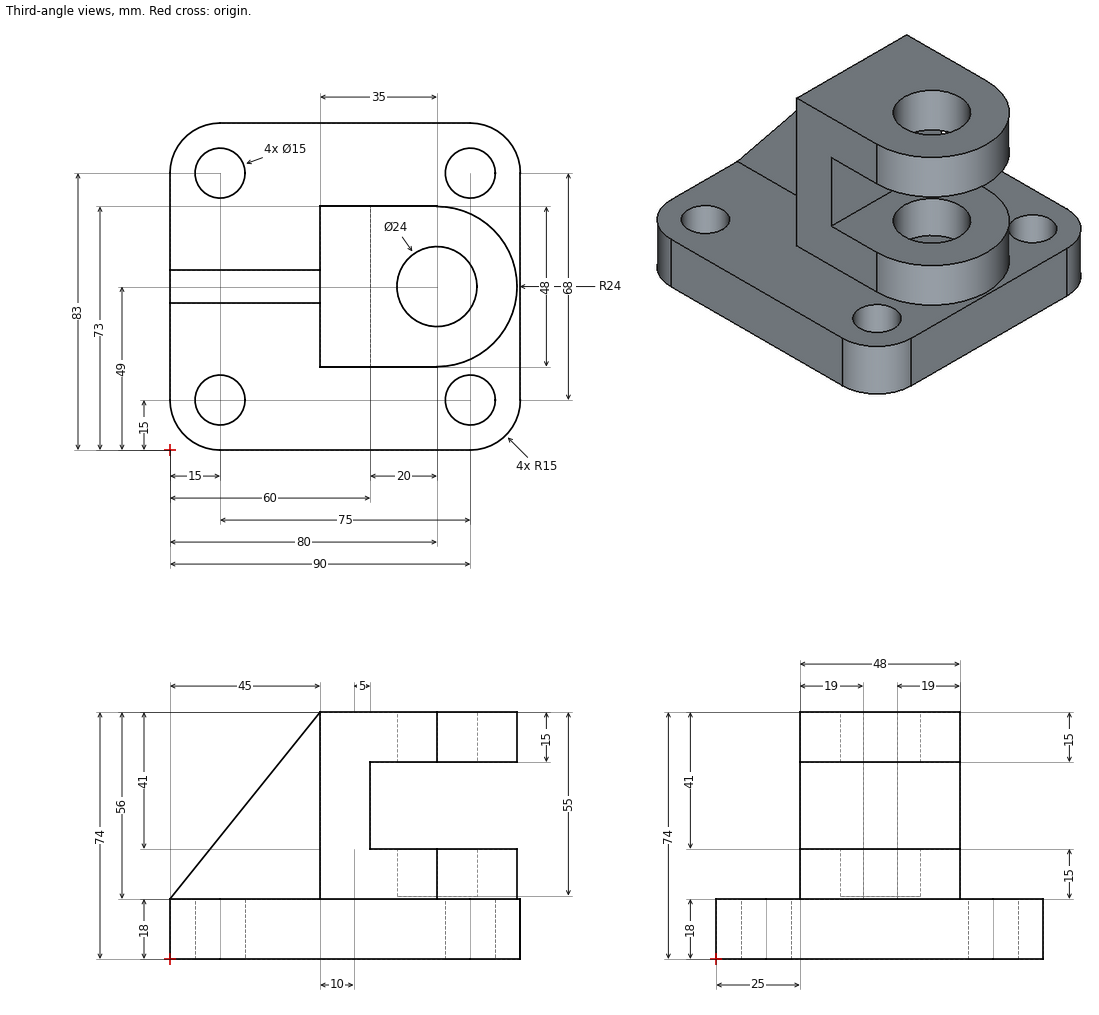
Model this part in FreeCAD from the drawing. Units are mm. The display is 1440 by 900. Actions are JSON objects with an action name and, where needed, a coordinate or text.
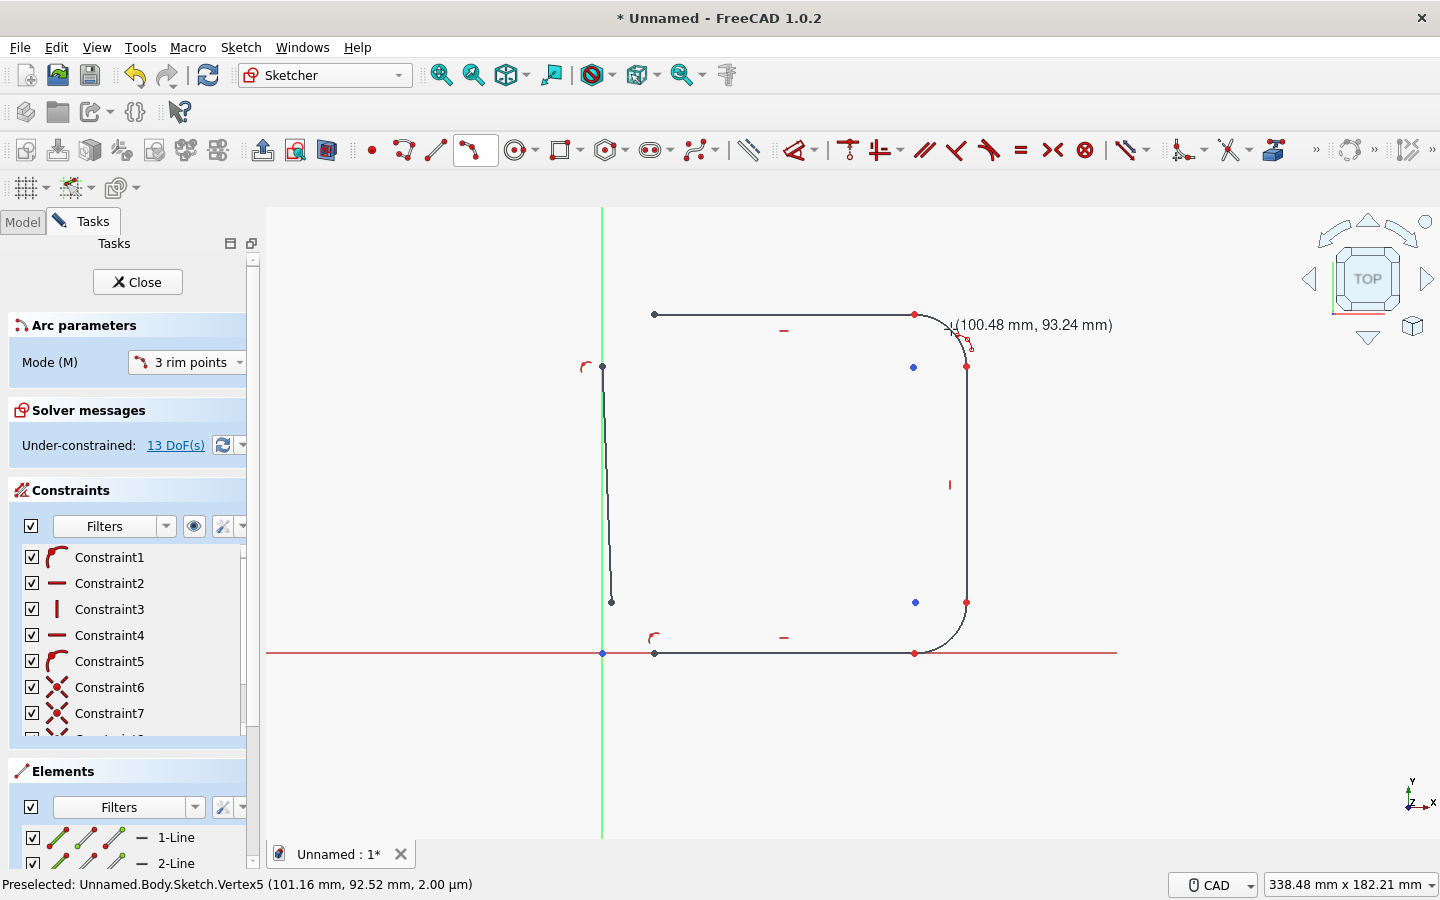
{"action": "left_click", "coordinate": [655, 315]}
{"action": "left_click", "coordinate": [602, 366]}
{"action": "left_click", "coordinate": [618, 329]}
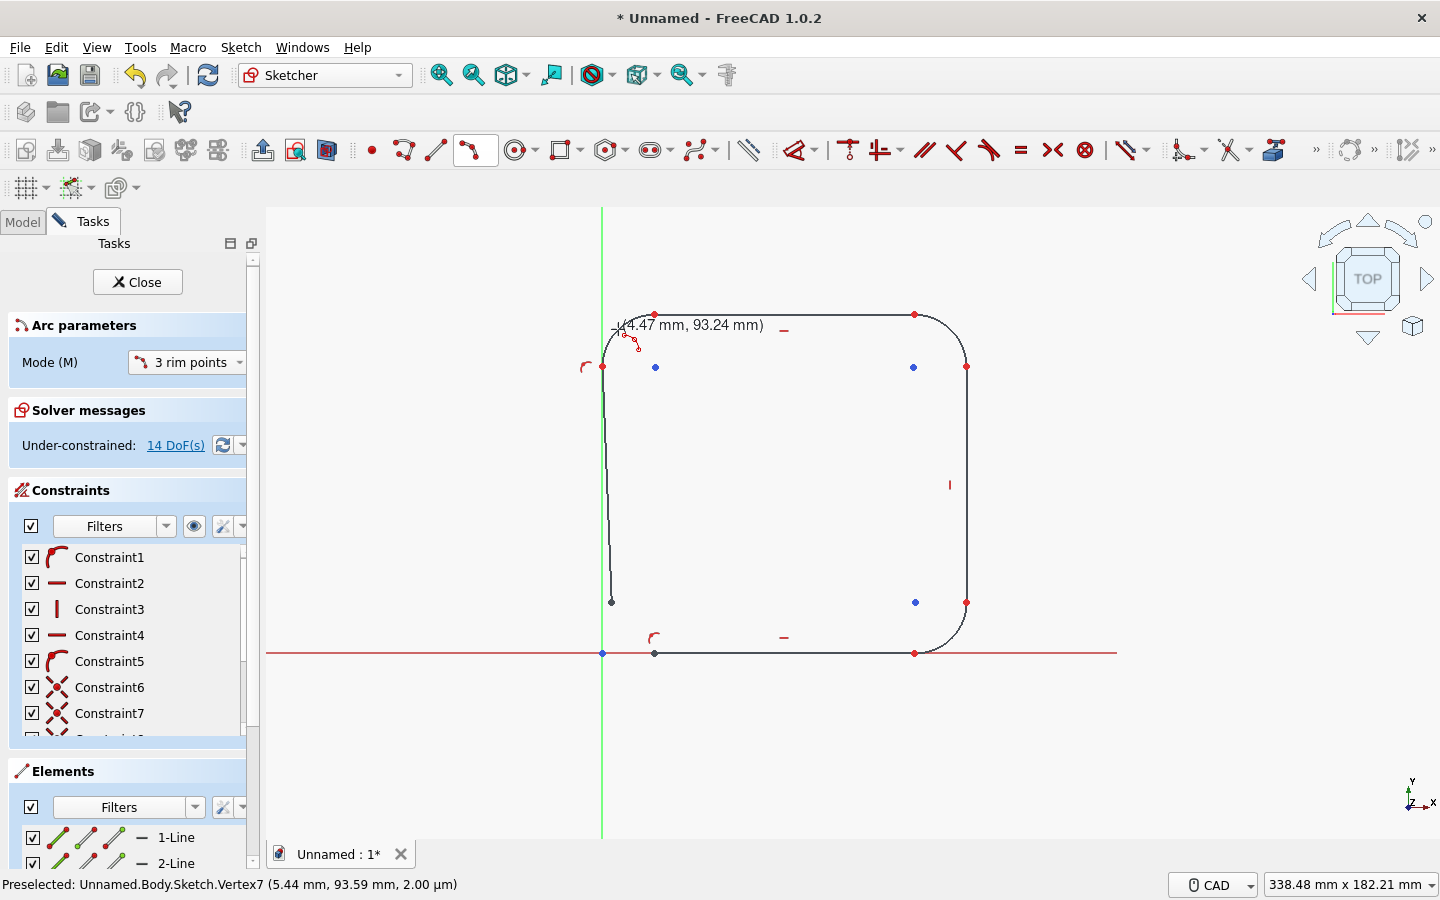
{"action": "left_click", "coordinate": [612, 603]}
{"action": "left_click", "coordinate": [655, 653]}
{"action": "left_click", "coordinate": [618, 638]}
{"action": "key", "text": "Escape"}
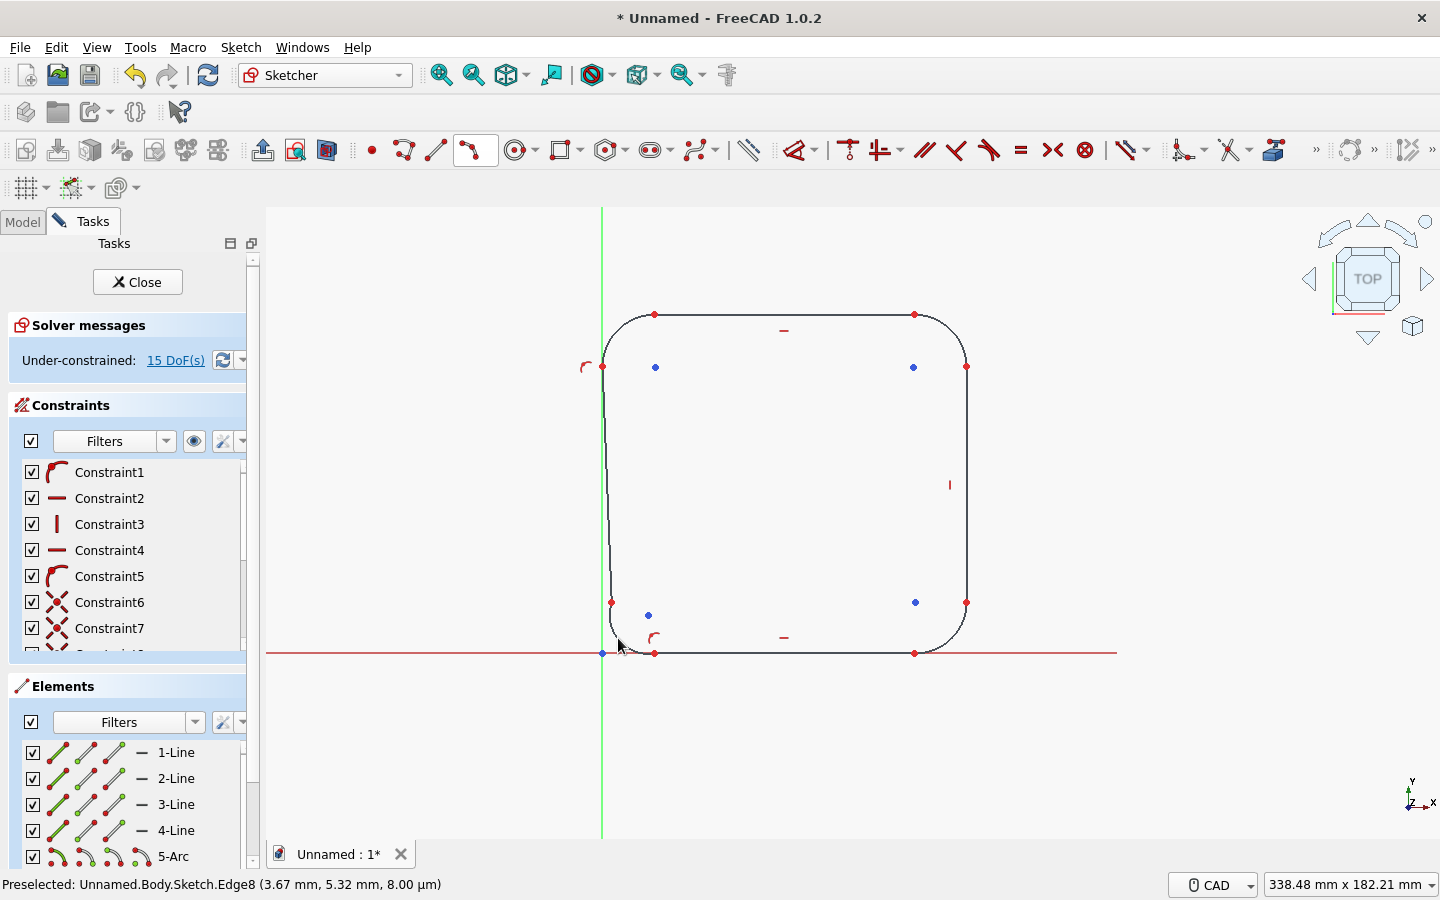
{"action": "left_click", "coordinate": [733, 653]}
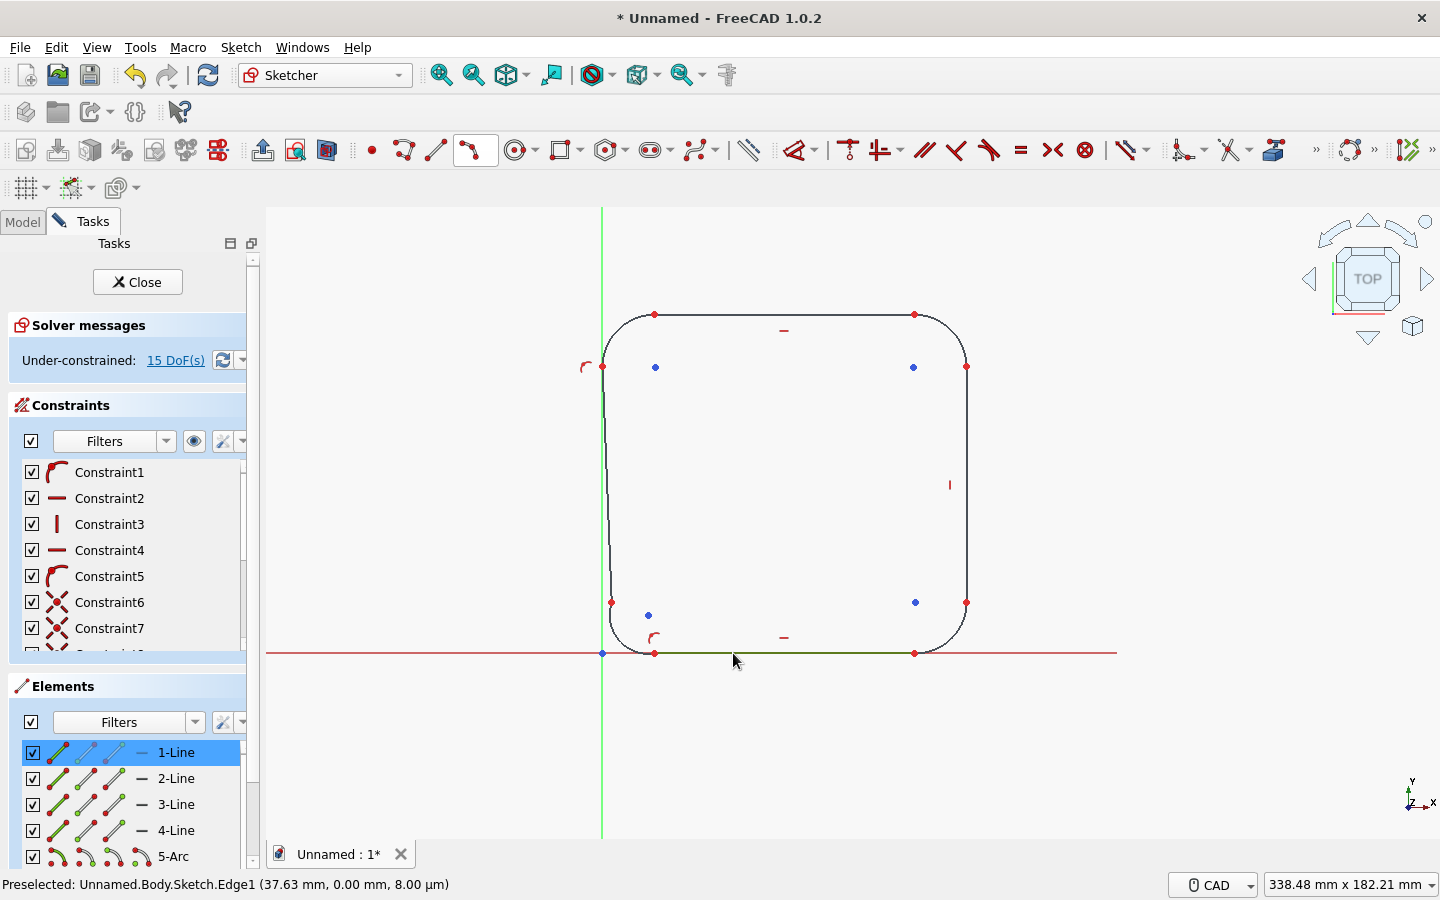
{"action": "left_click", "coordinate": [961, 626]}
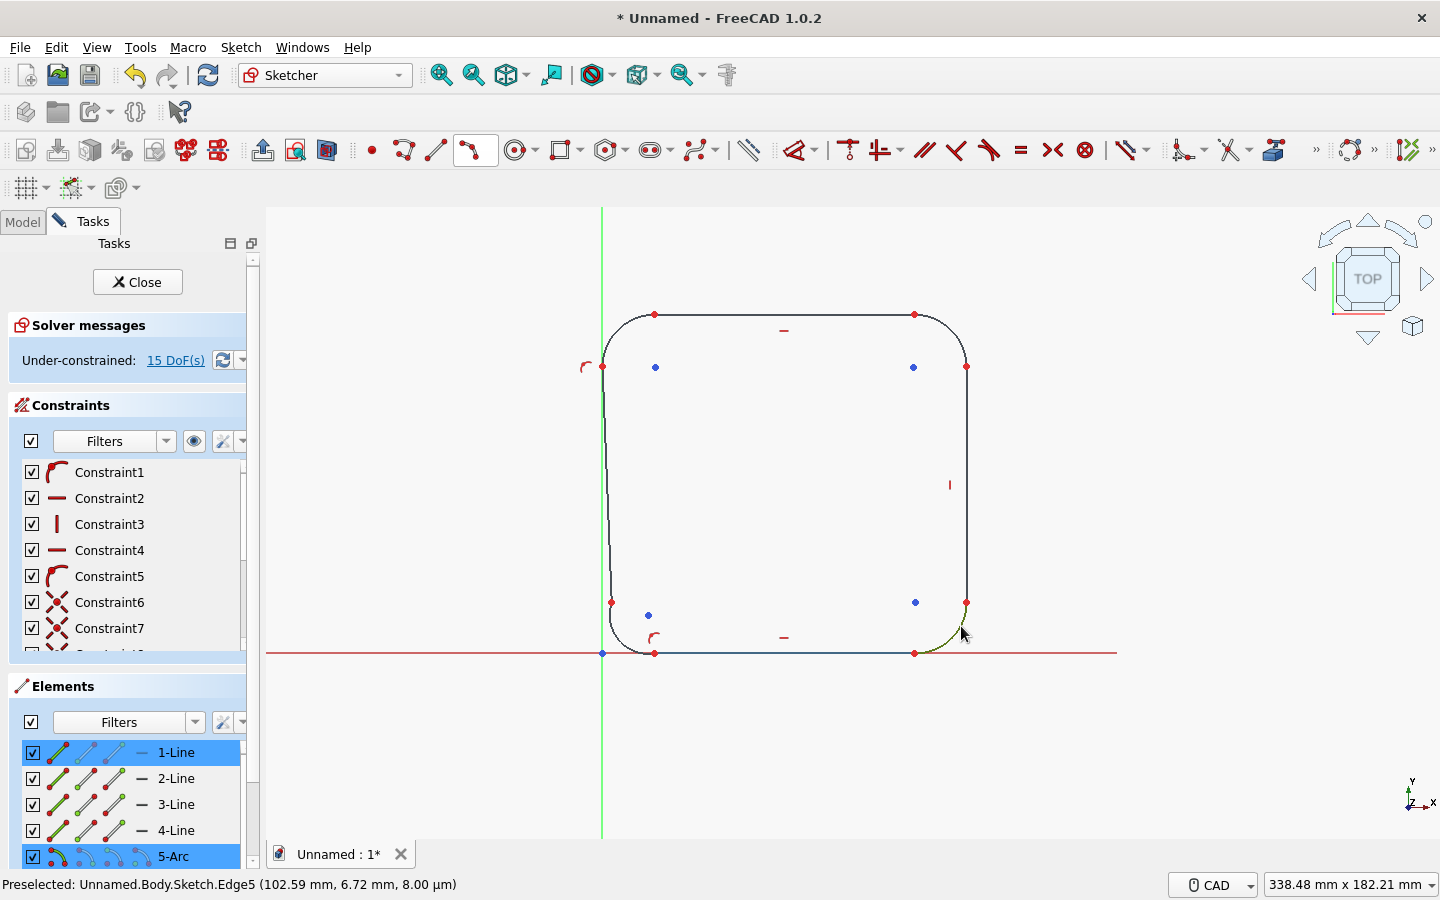
{"action": "left_click", "coordinate": [990, 150]}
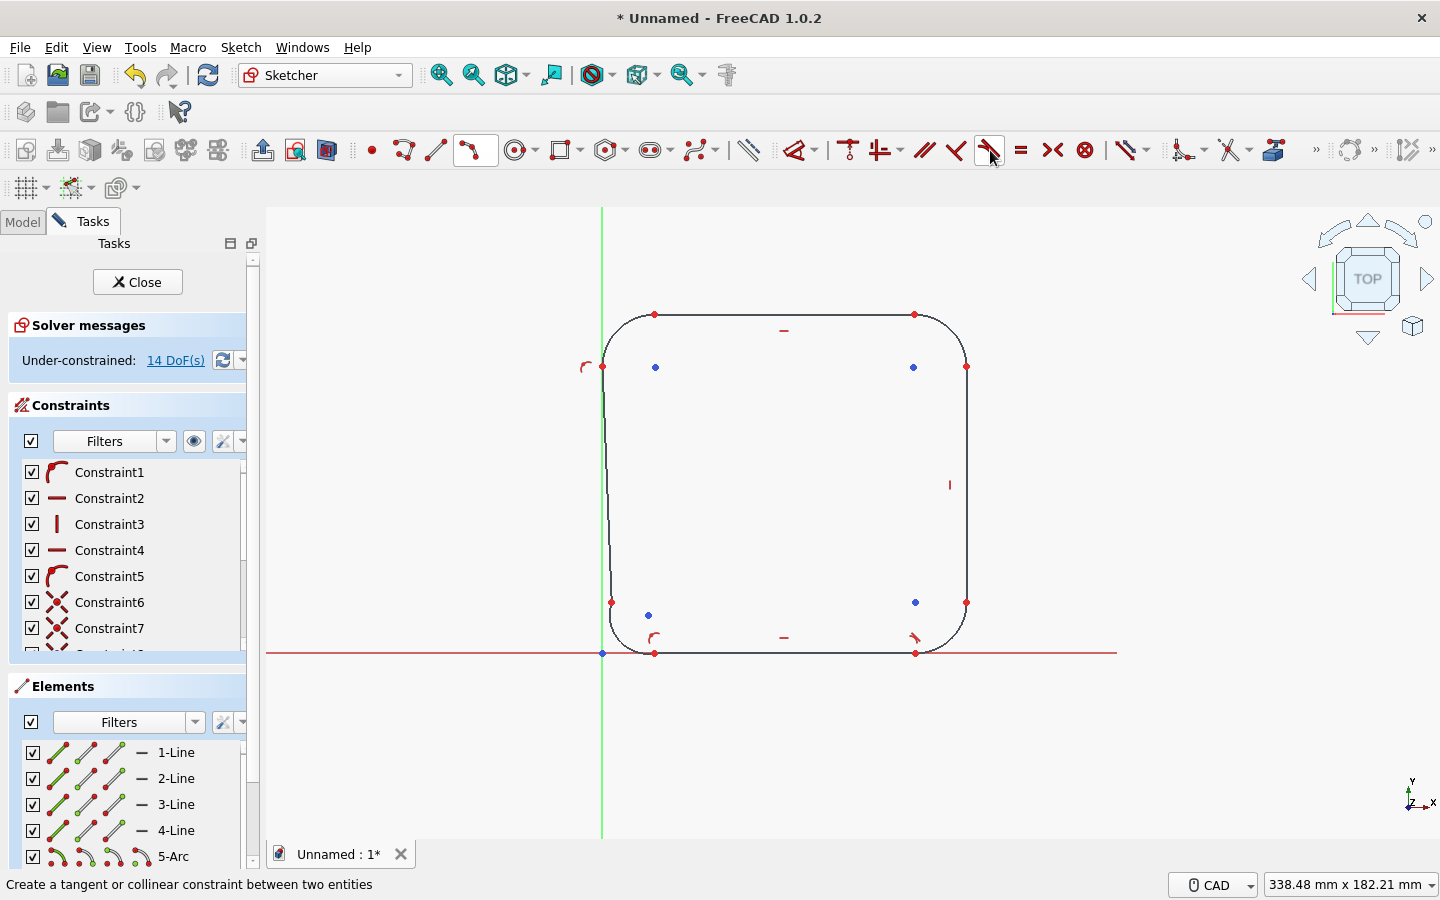
{"action": "left_click", "coordinate": [733, 653]}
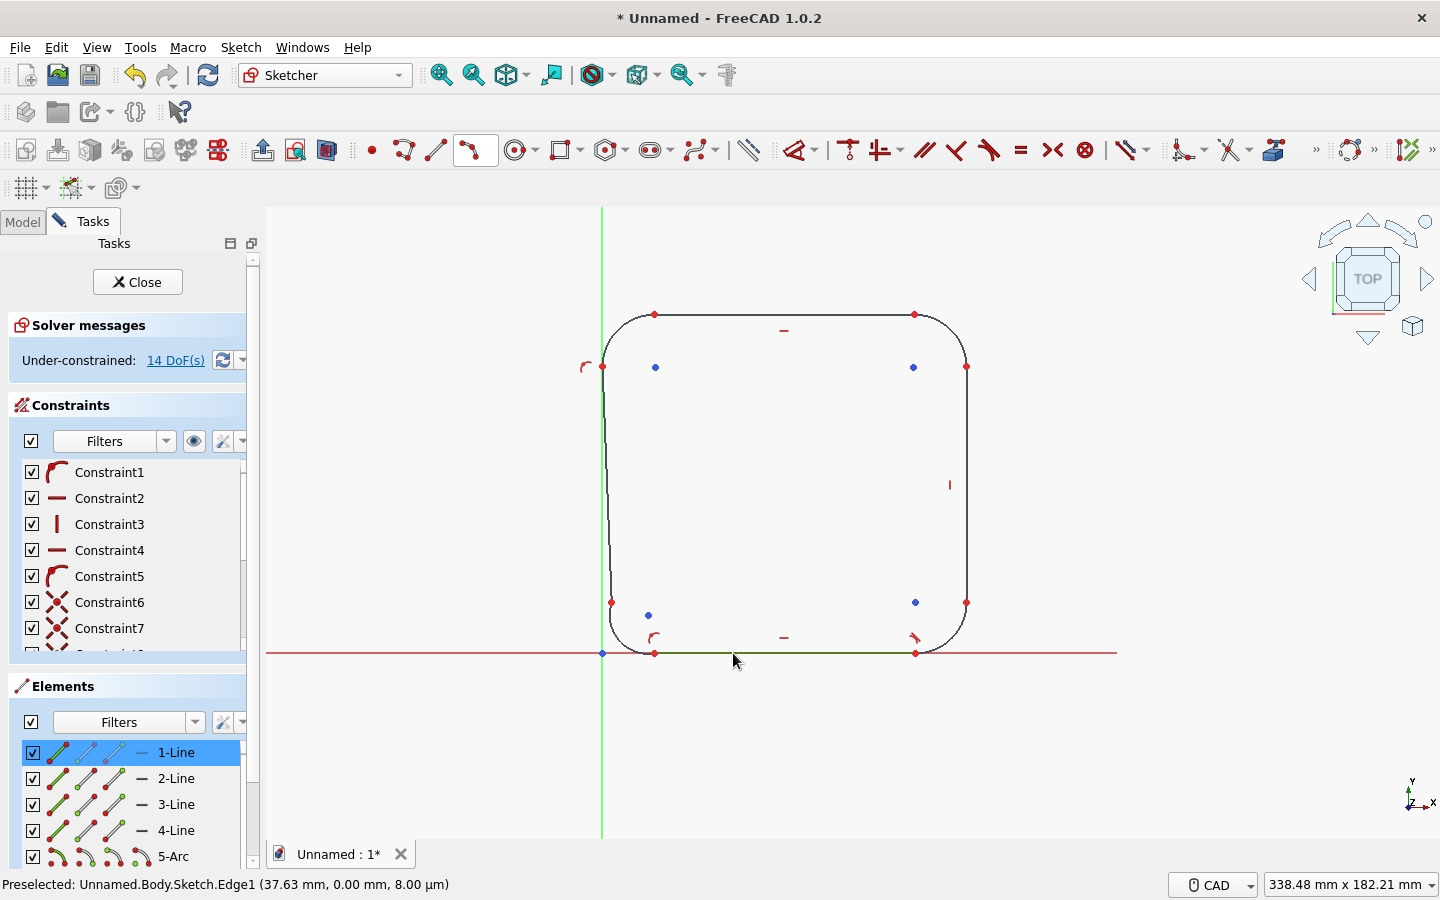
{"action": "left_click", "coordinate": [631, 650]}